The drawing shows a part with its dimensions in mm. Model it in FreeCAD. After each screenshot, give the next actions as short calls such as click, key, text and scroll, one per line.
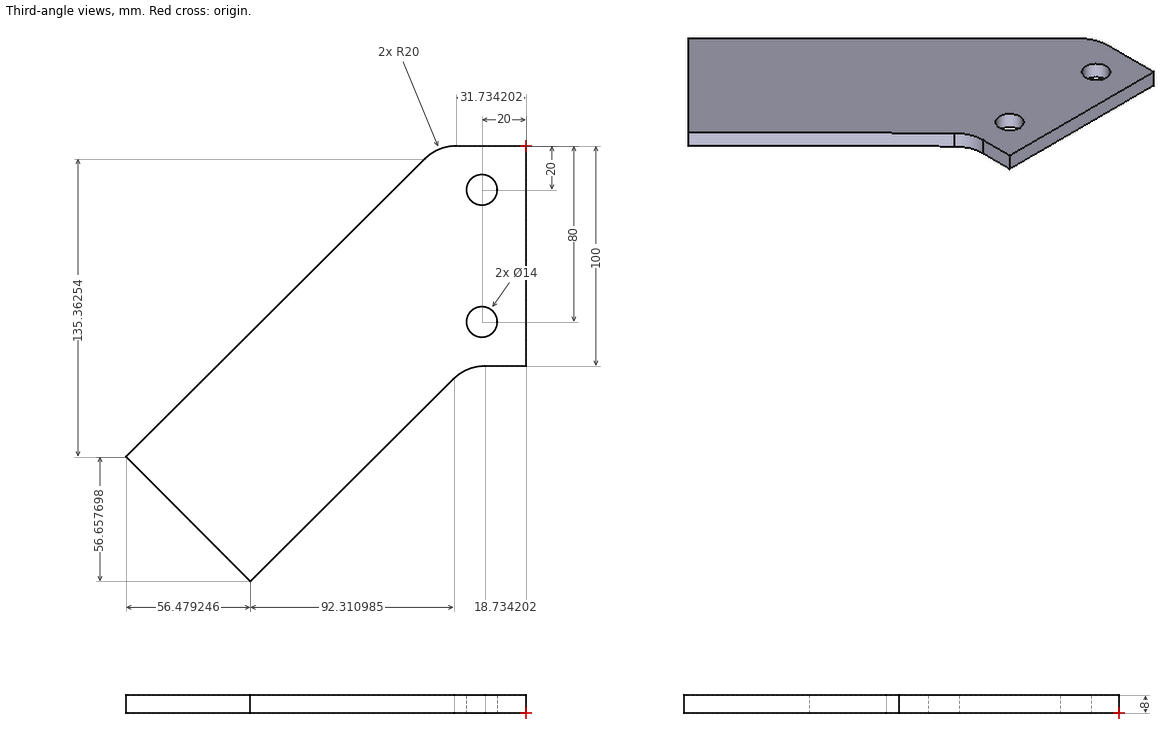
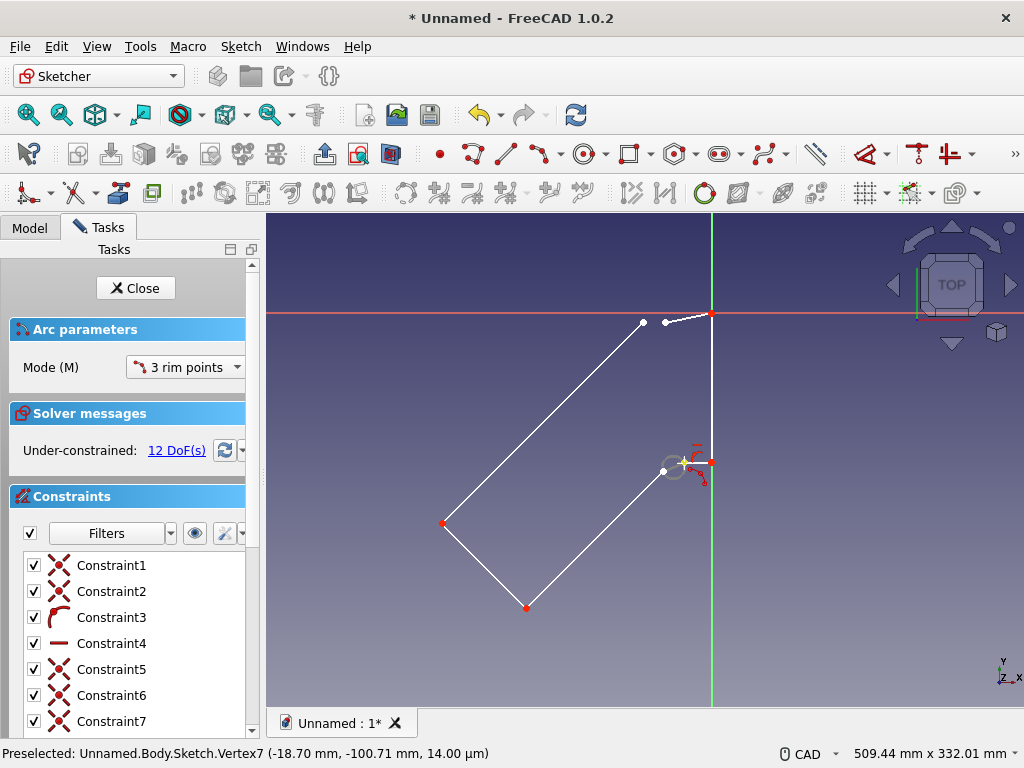
scroll(673, 464, up, 10)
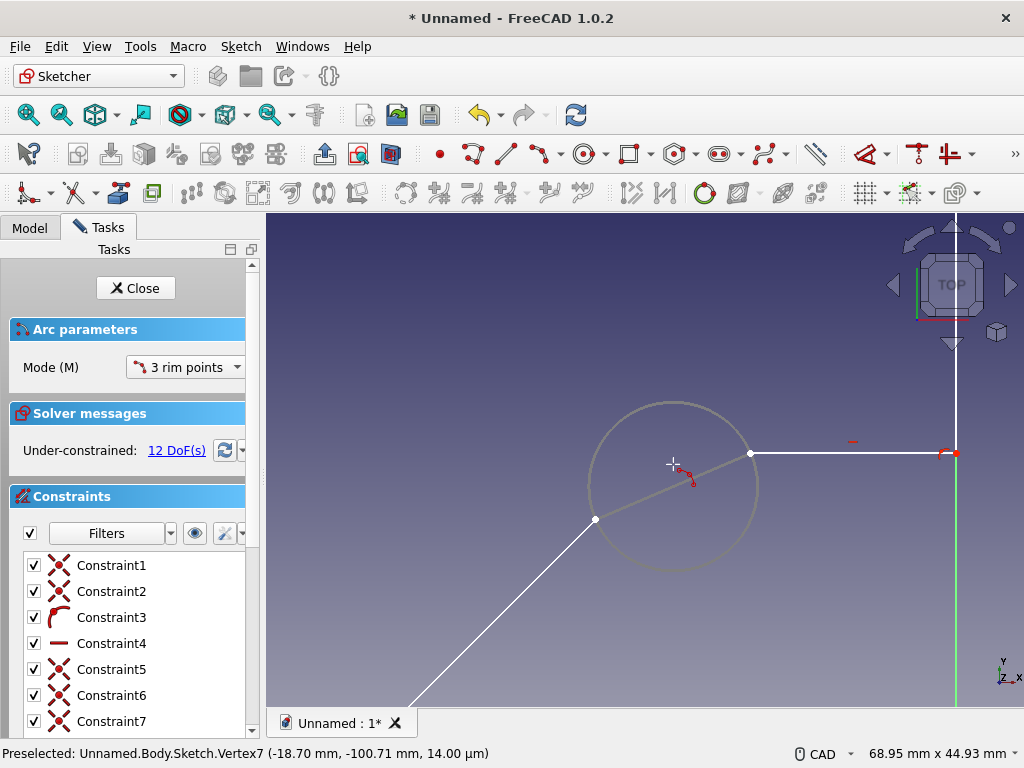
click(666, 462)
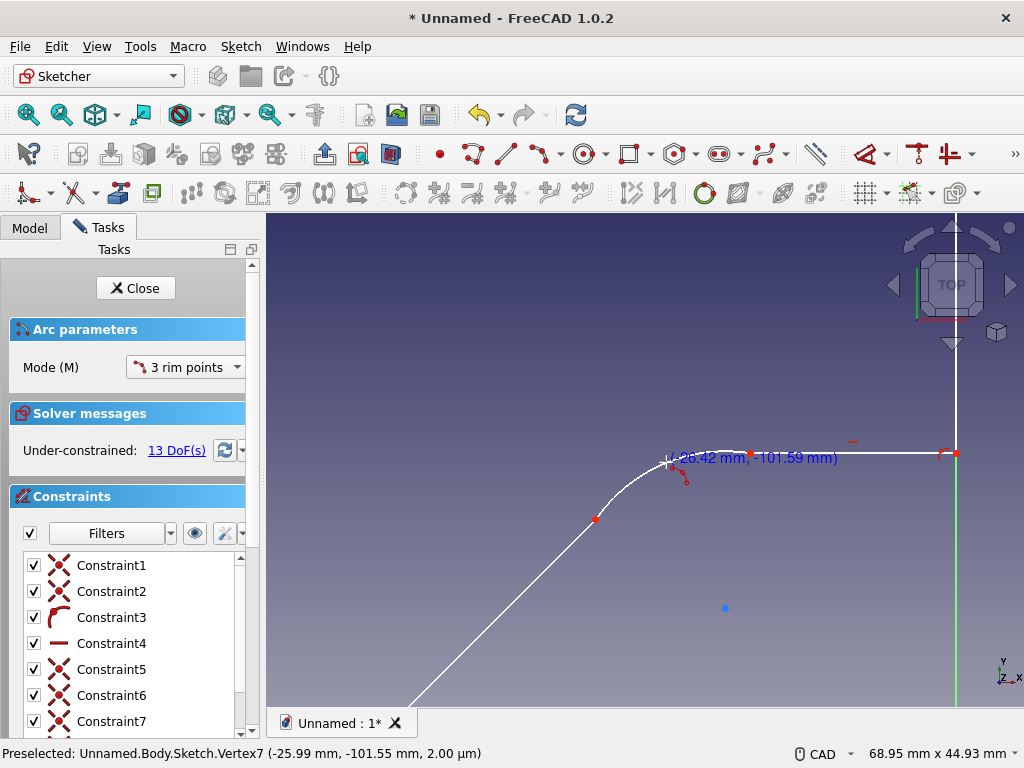
scroll(673, 464, down, 10)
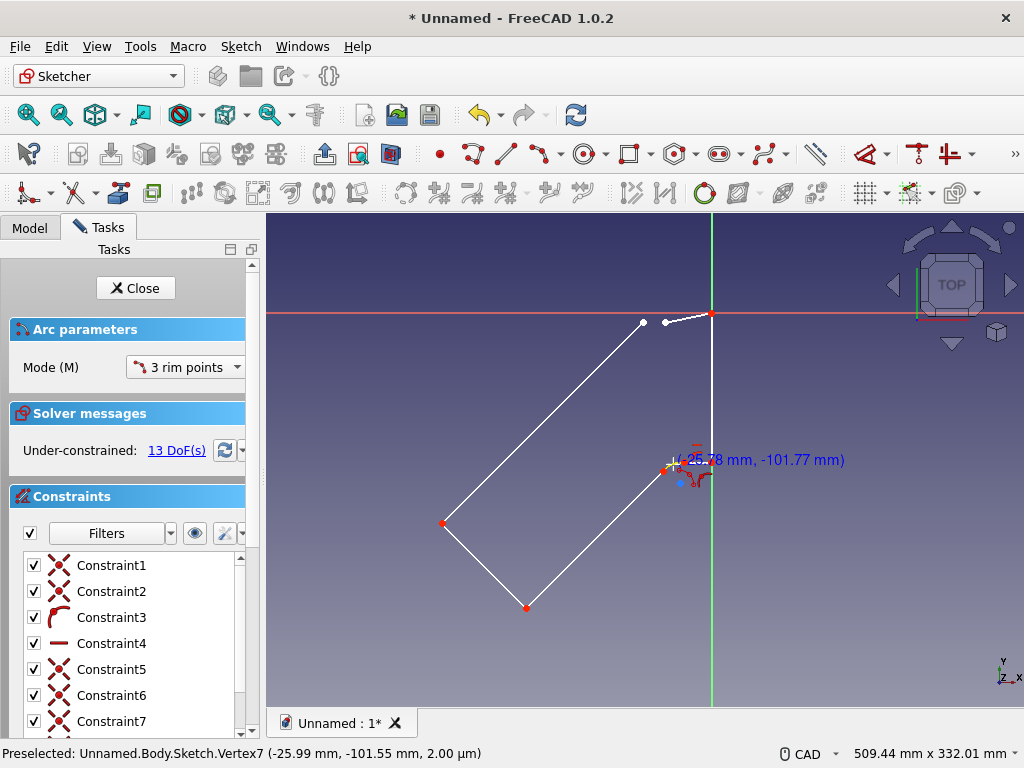
click(665, 323)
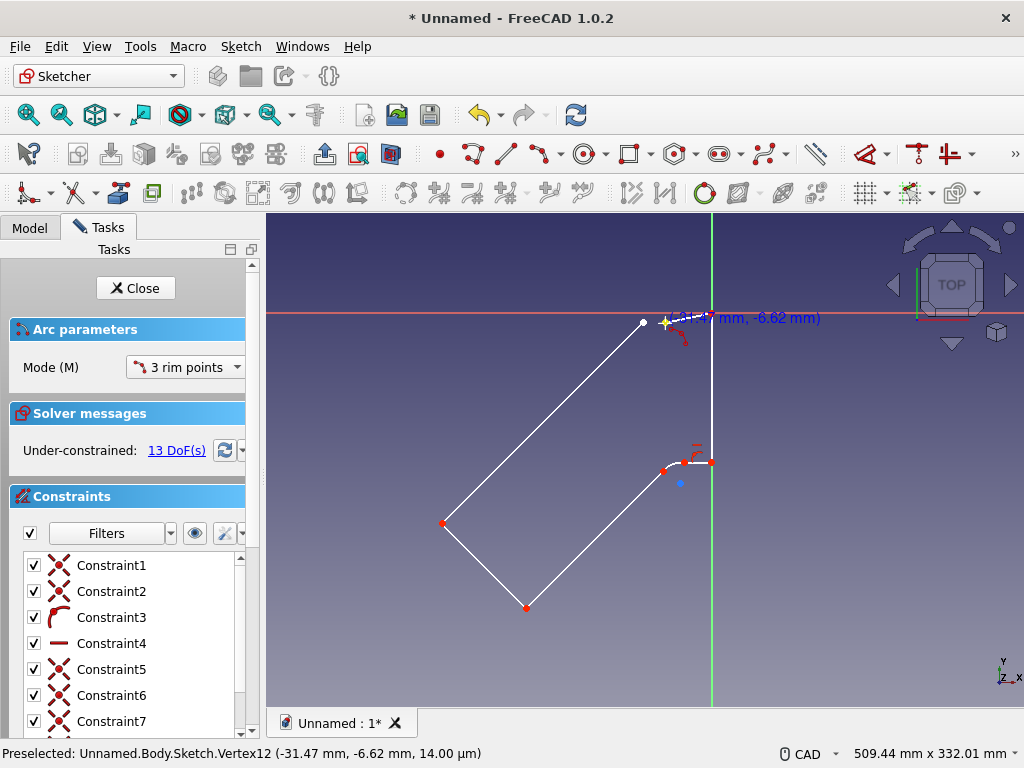
scroll(644, 322, up, 4)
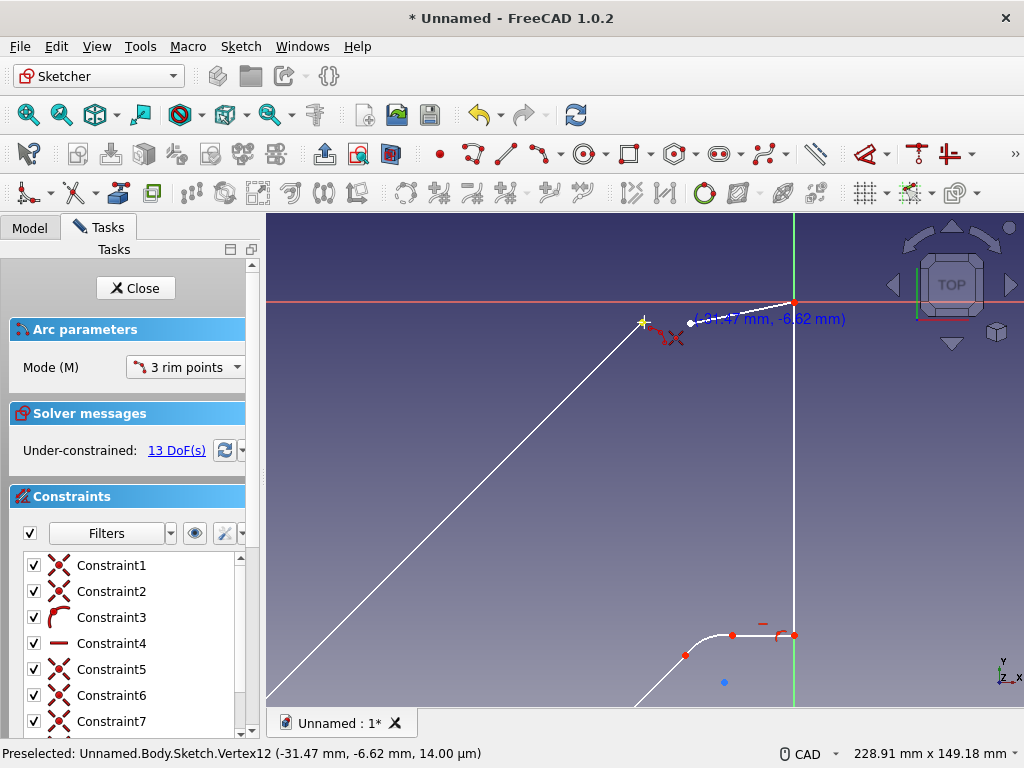
click(642, 322)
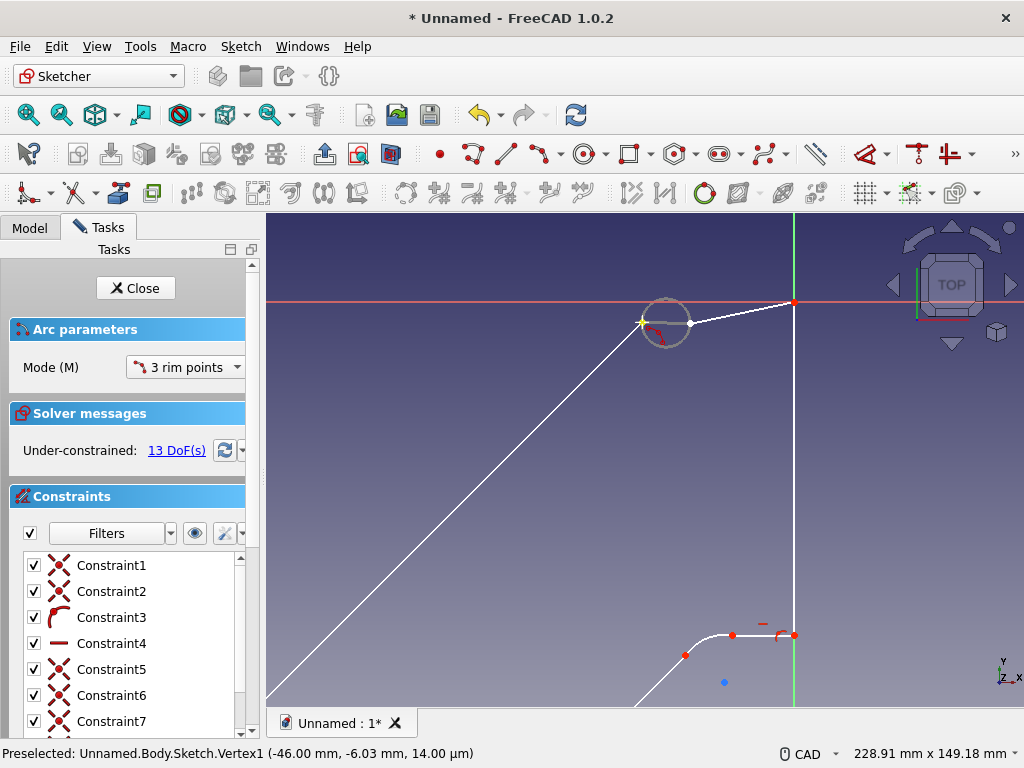
scroll(664, 307, up, 6)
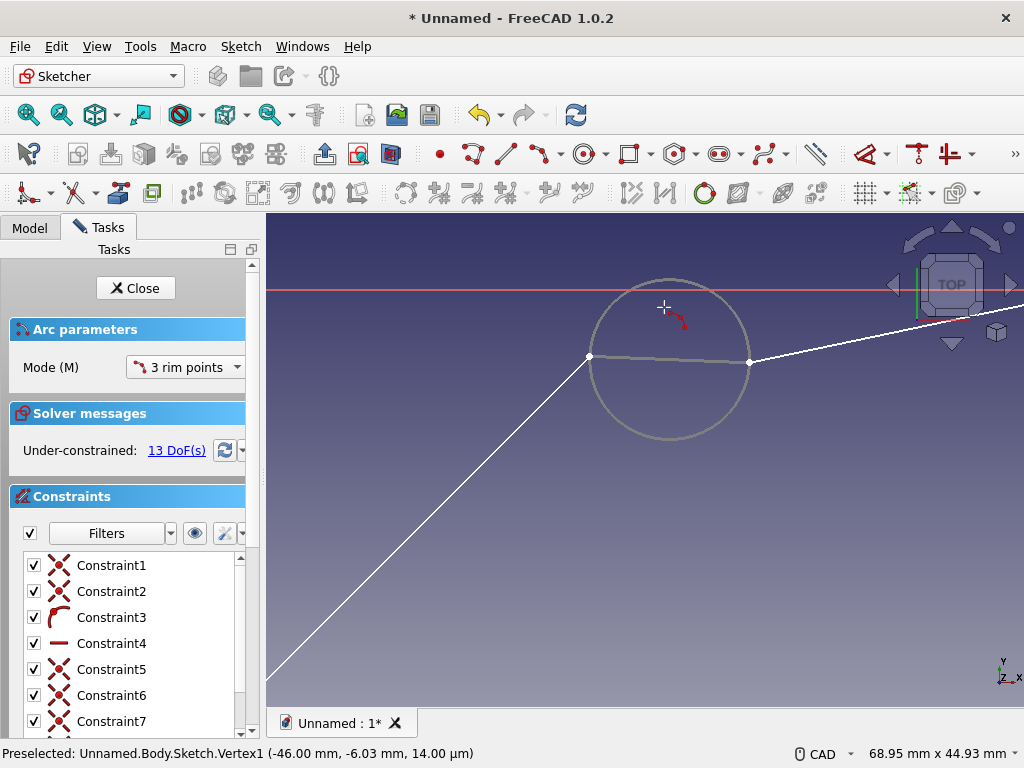
click(663, 307)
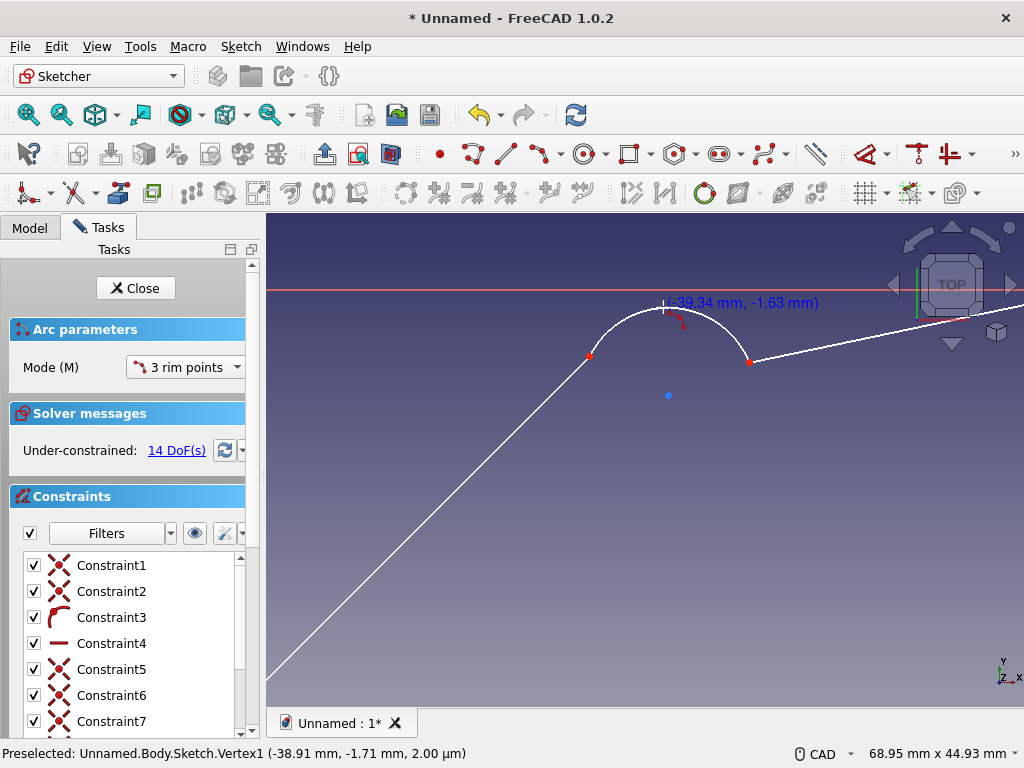
click(584, 154)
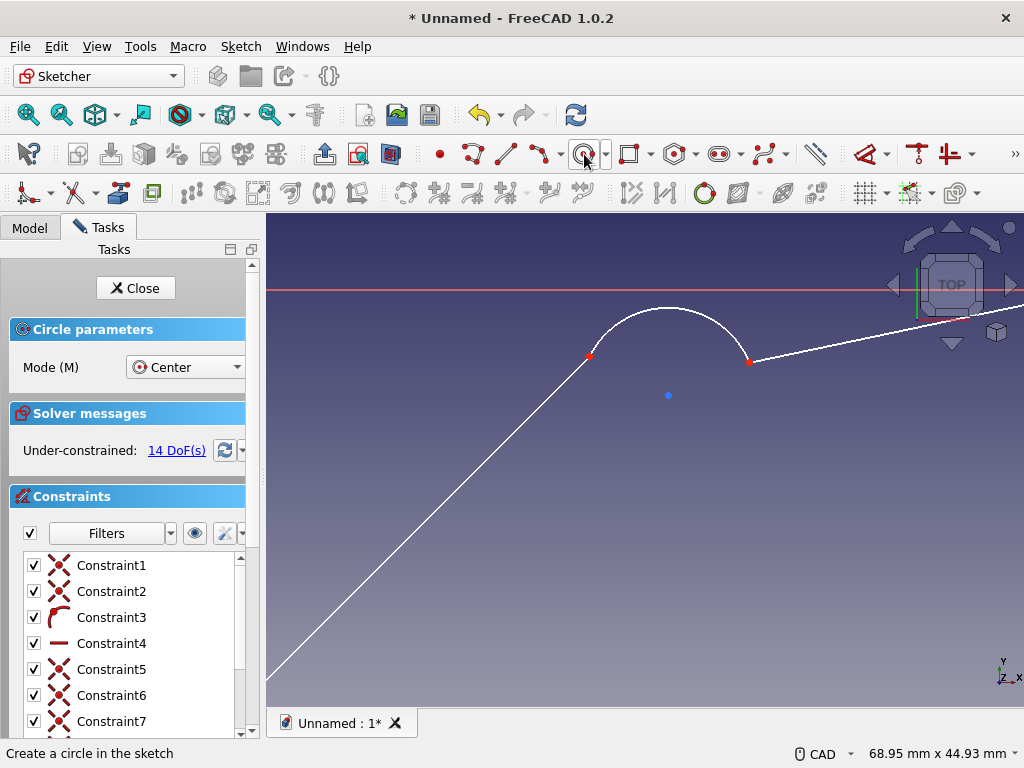
scroll(652, 316, down, 10)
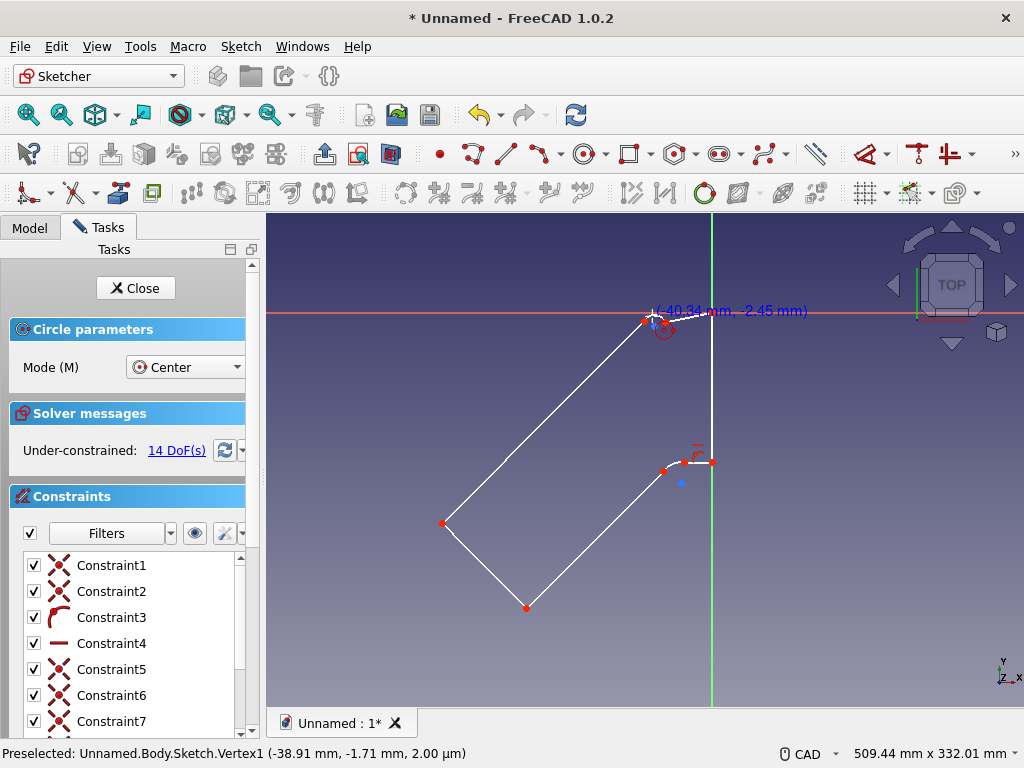
scroll(683, 432, up, 4)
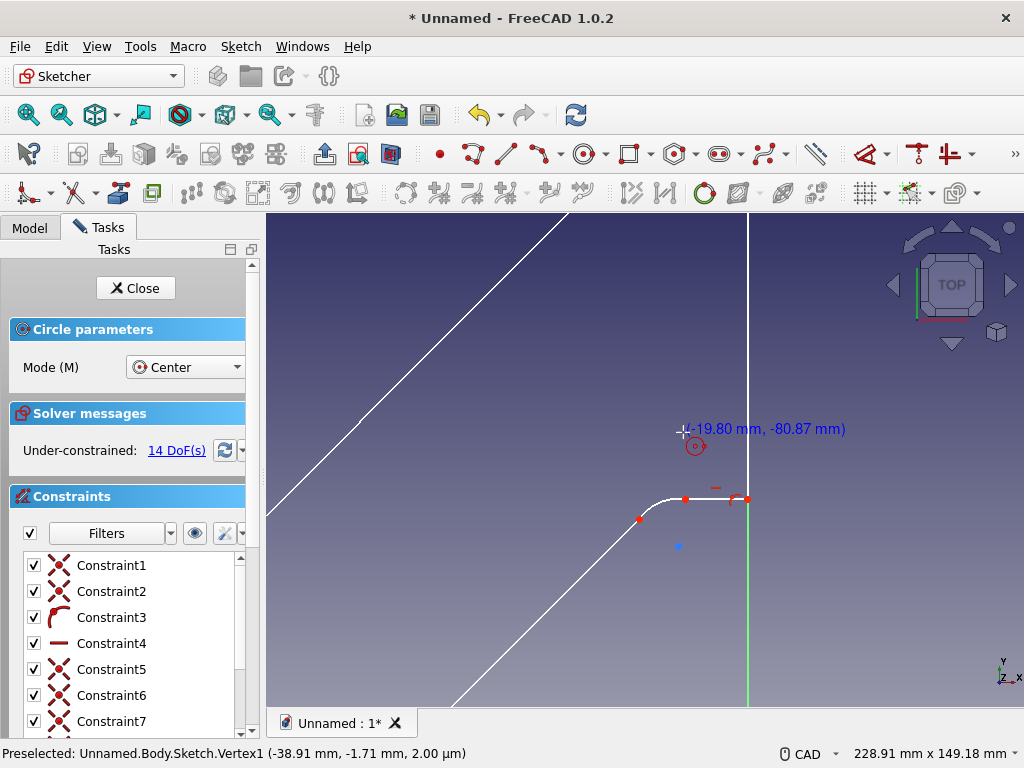
click(682, 431)
click(698, 414)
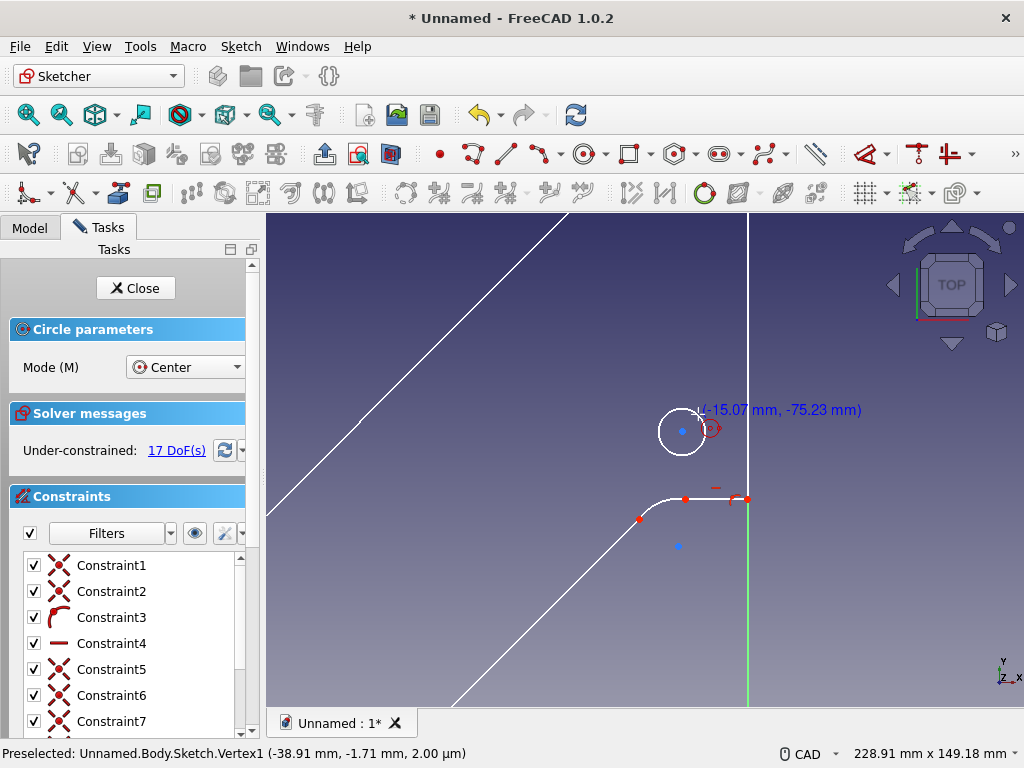
scroll(682, 433, down, 4)